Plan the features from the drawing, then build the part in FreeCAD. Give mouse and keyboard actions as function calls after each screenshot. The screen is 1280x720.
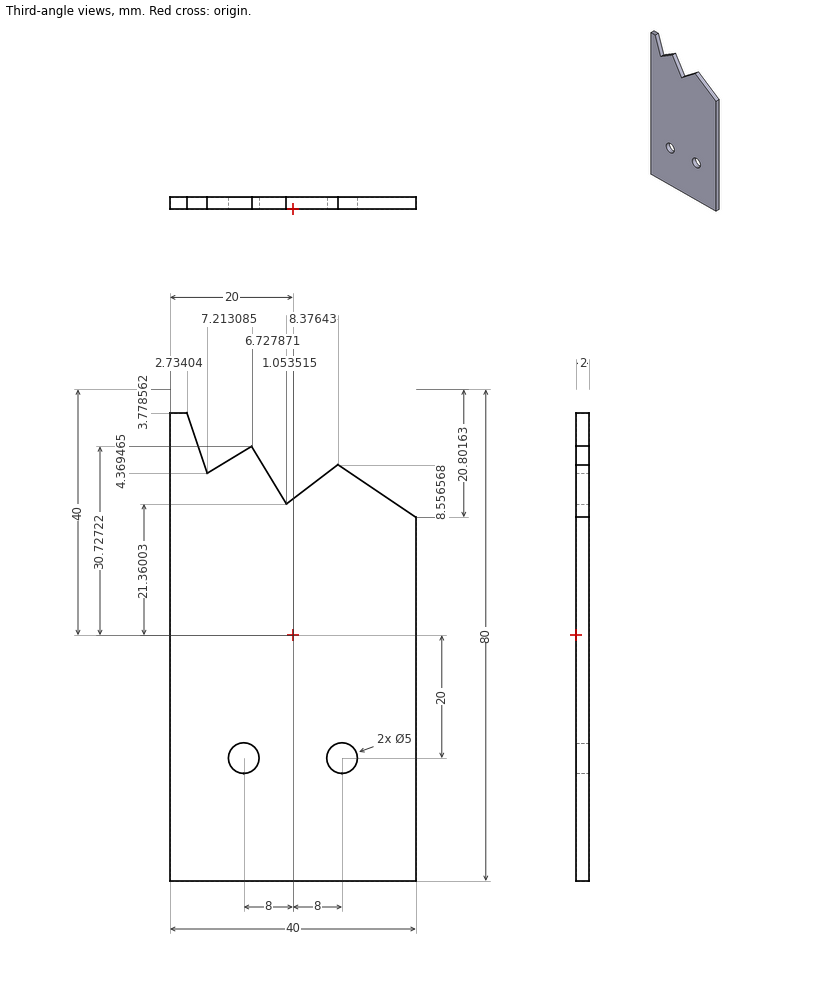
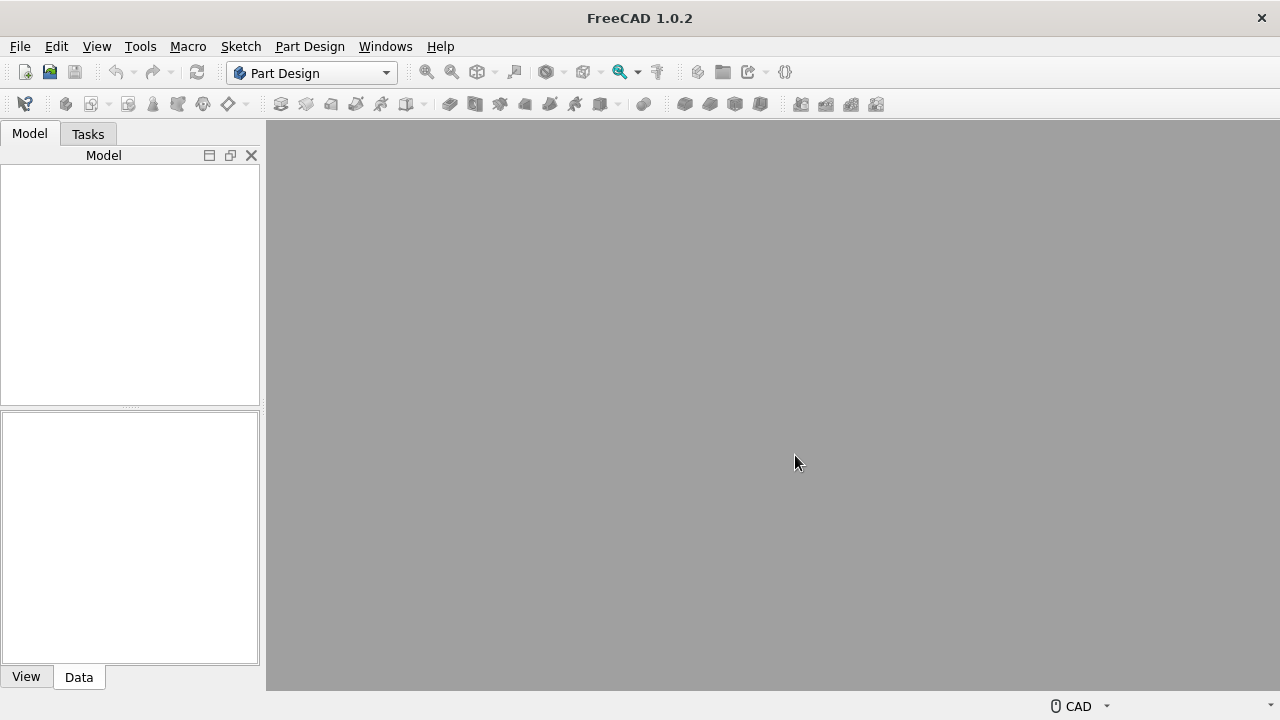
key(ctrl+n)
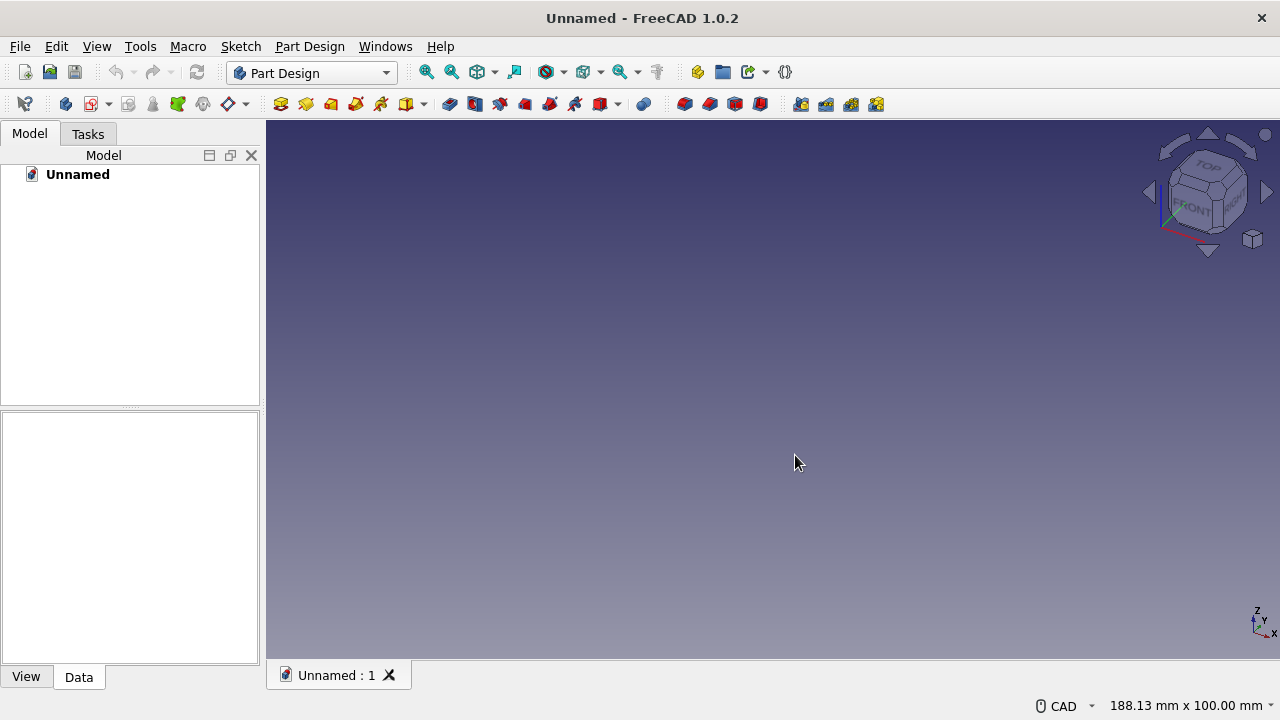
click(90, 104)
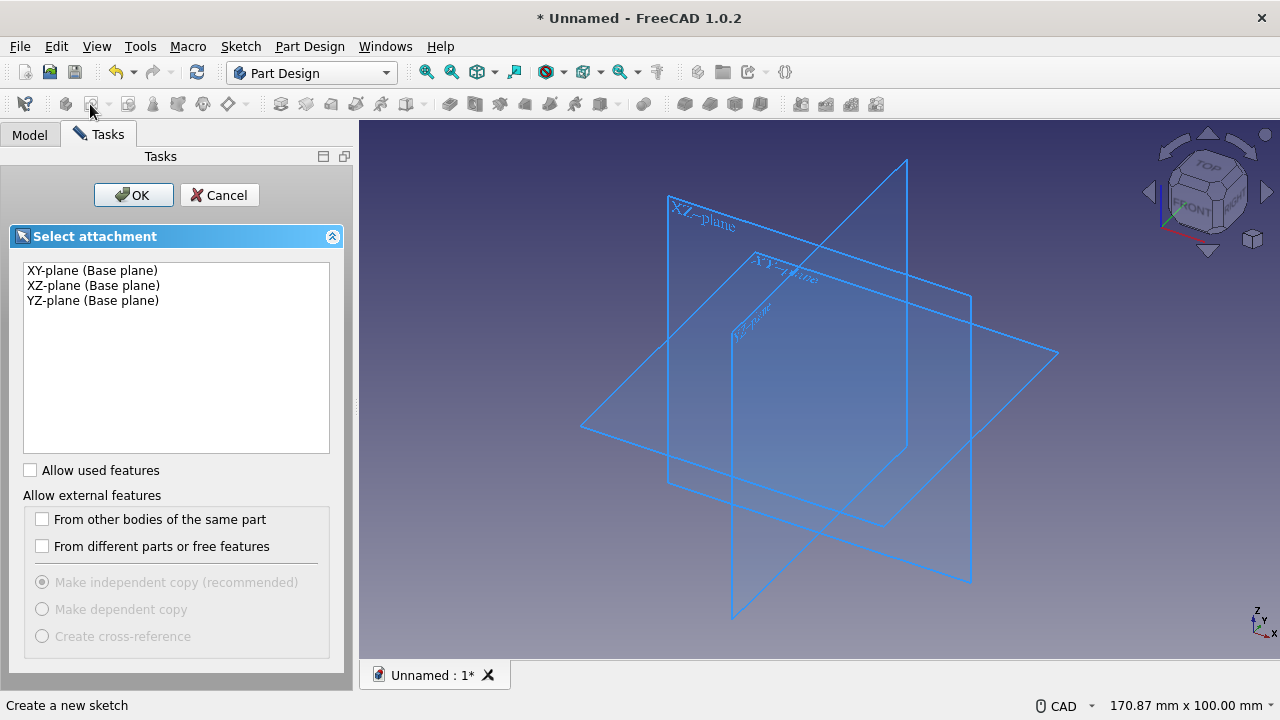
click(84, 286)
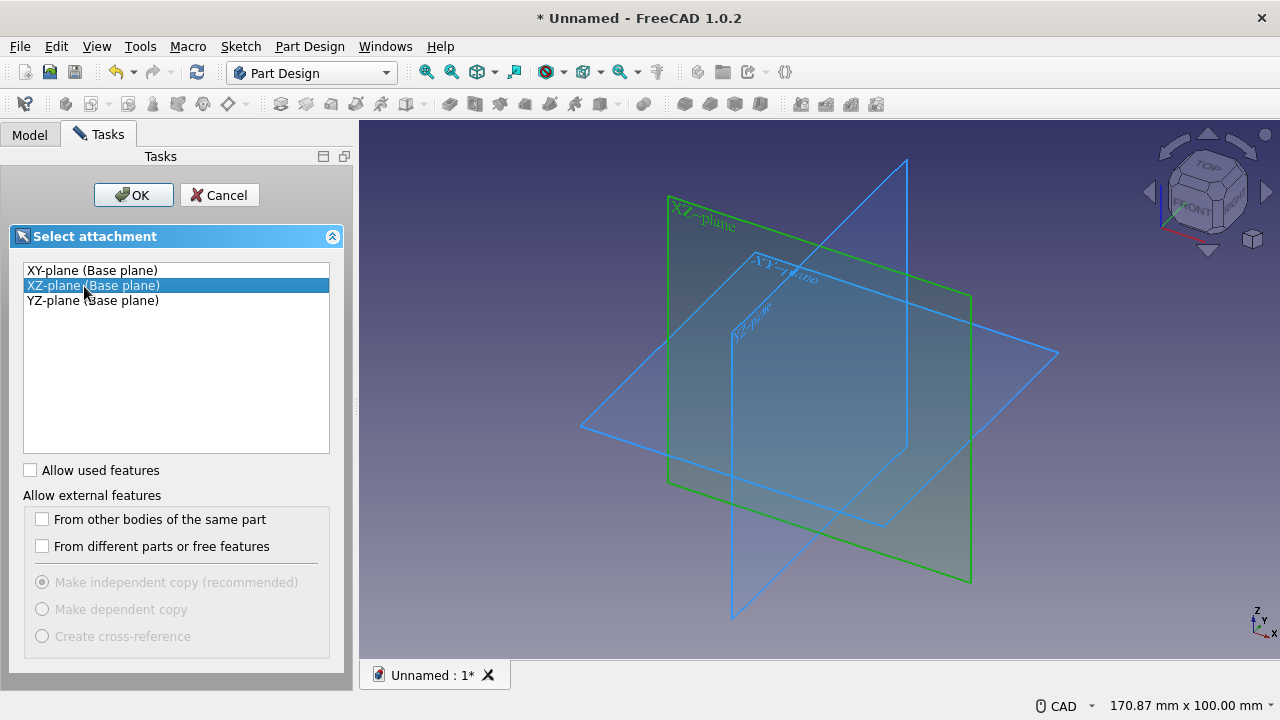
click(134, 195)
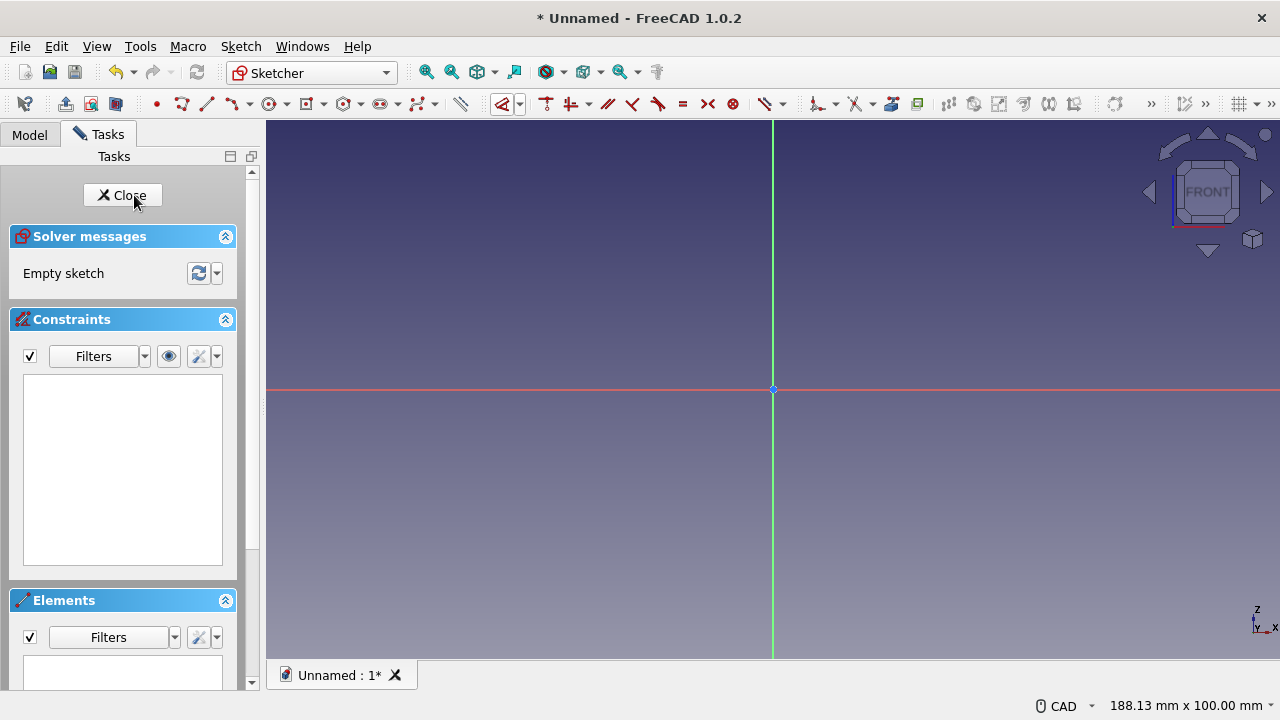
click(306, 104)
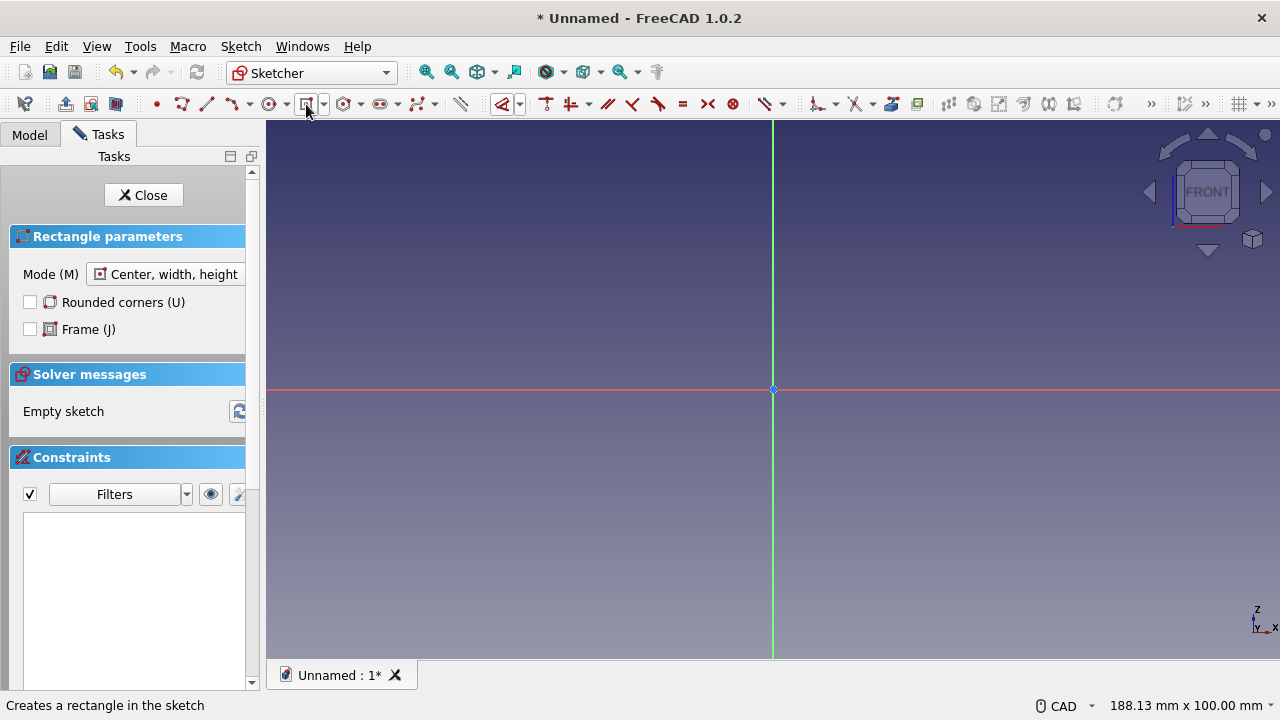
click(773, 390)
click(881, 174)
key(Escape)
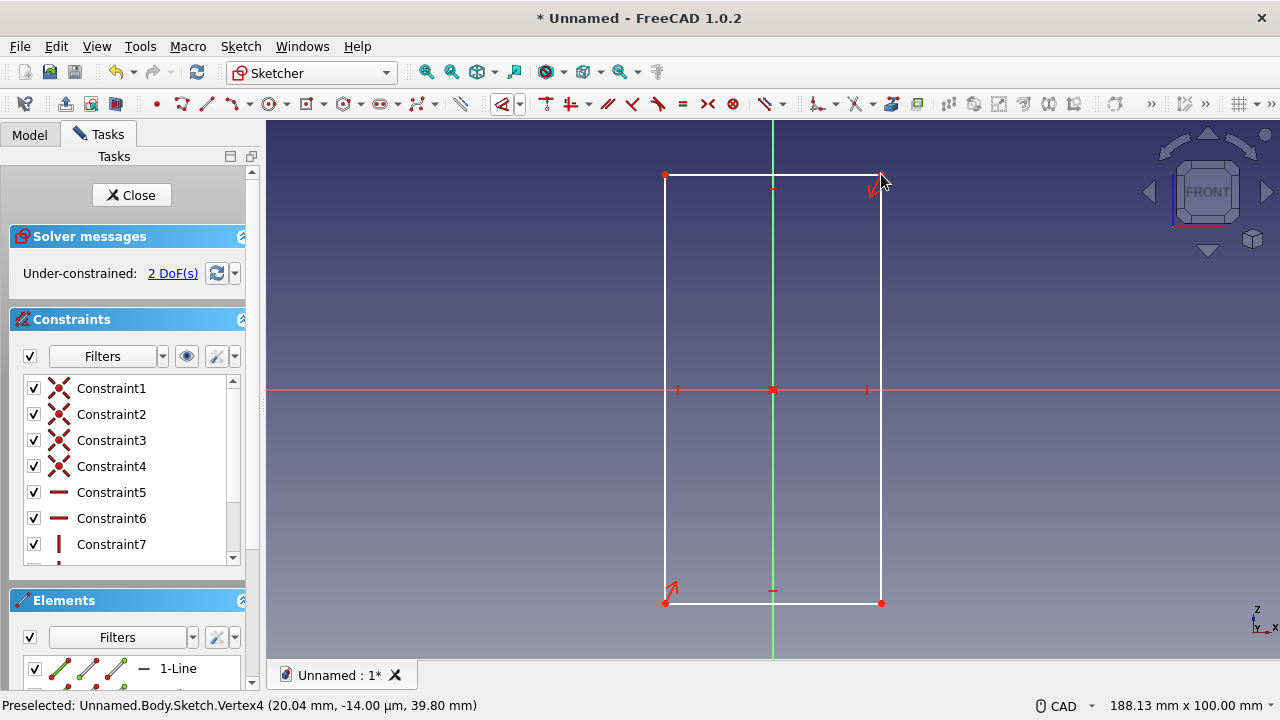
click(730, 604)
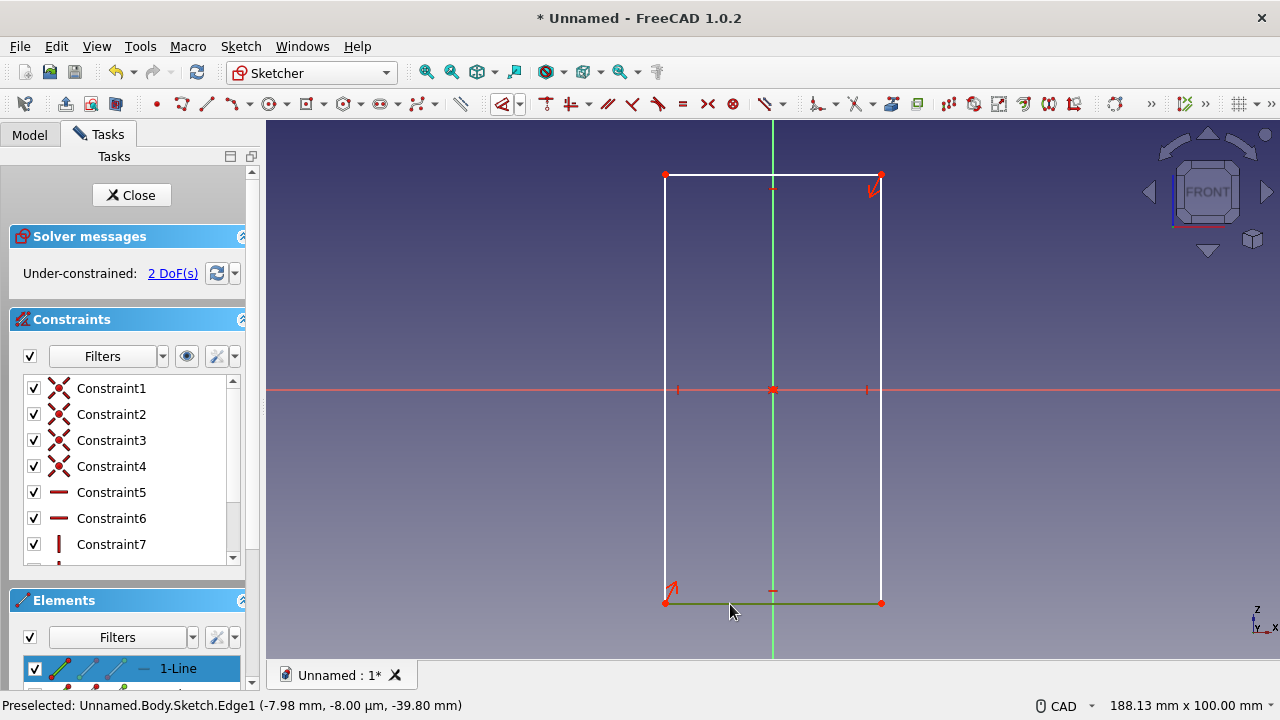
key(l)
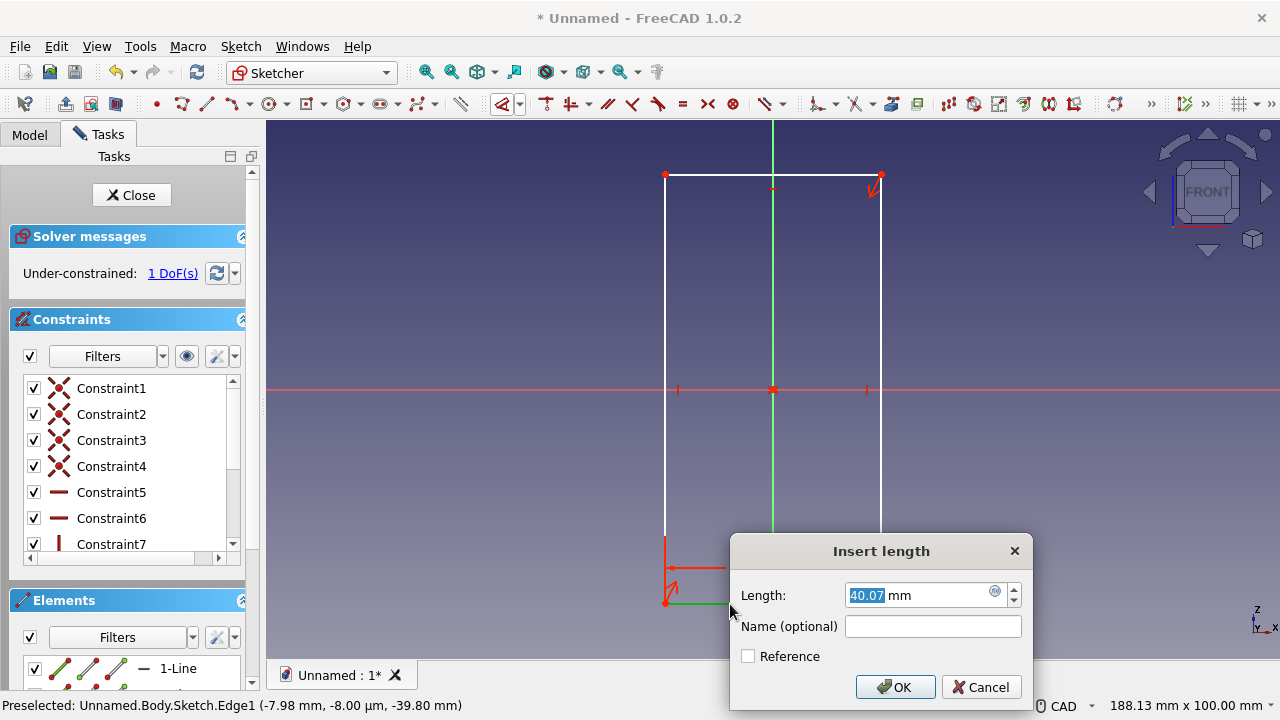
text(40)
key(Return)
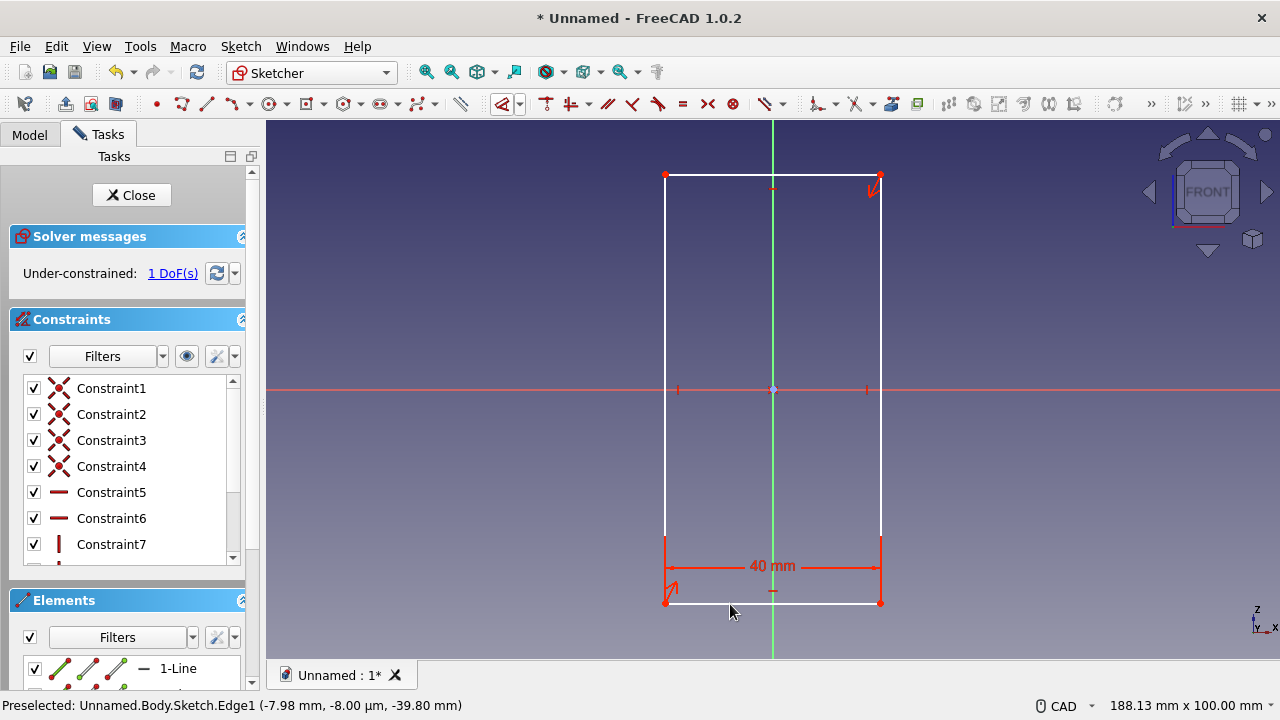
click(881, 475)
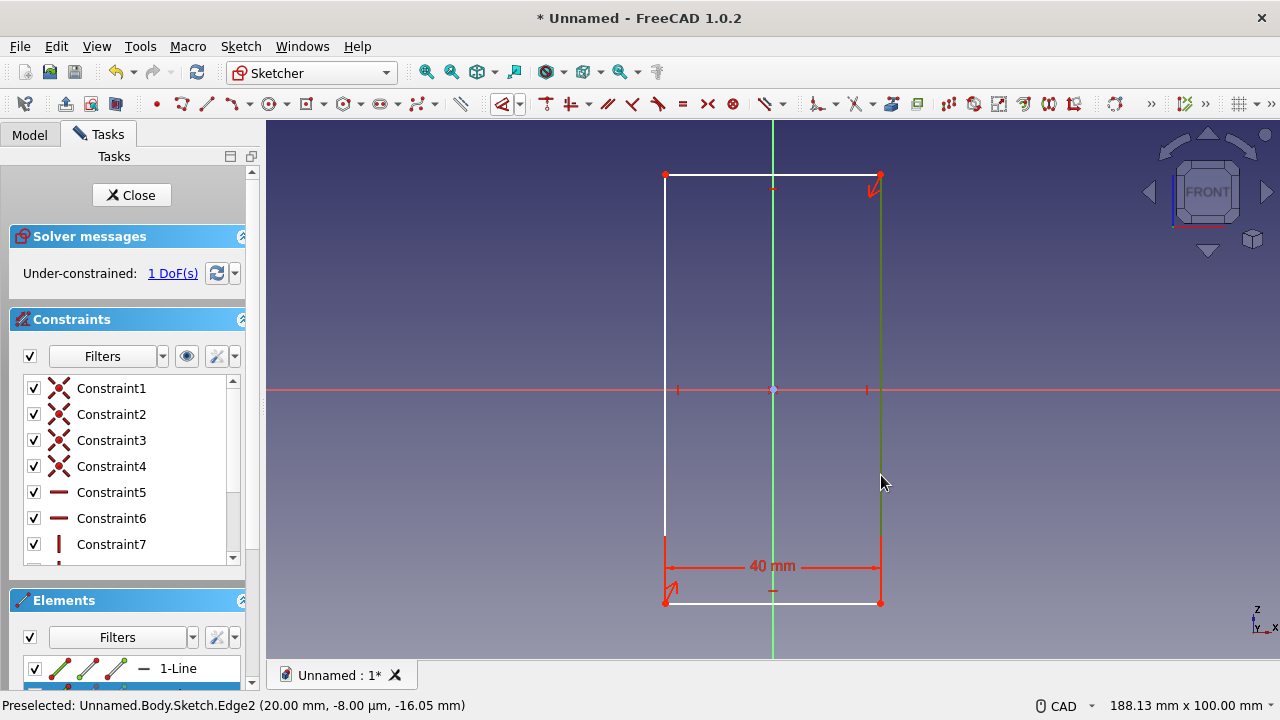
key(i)